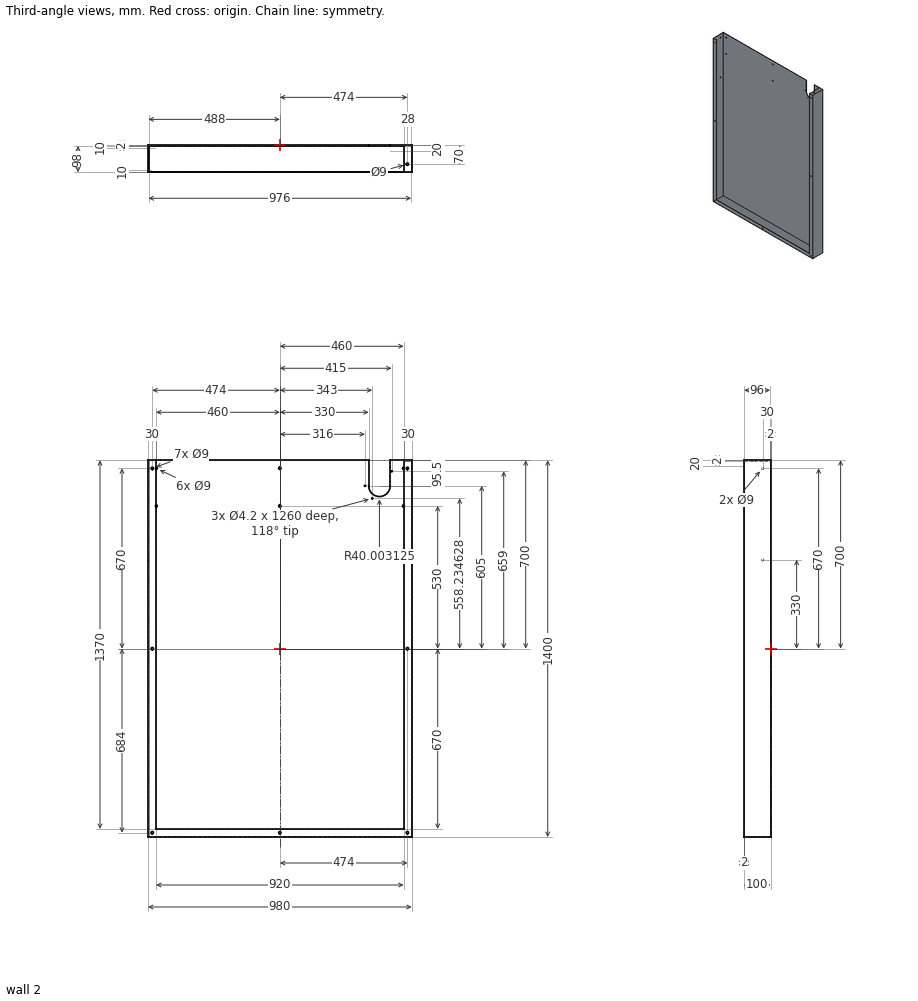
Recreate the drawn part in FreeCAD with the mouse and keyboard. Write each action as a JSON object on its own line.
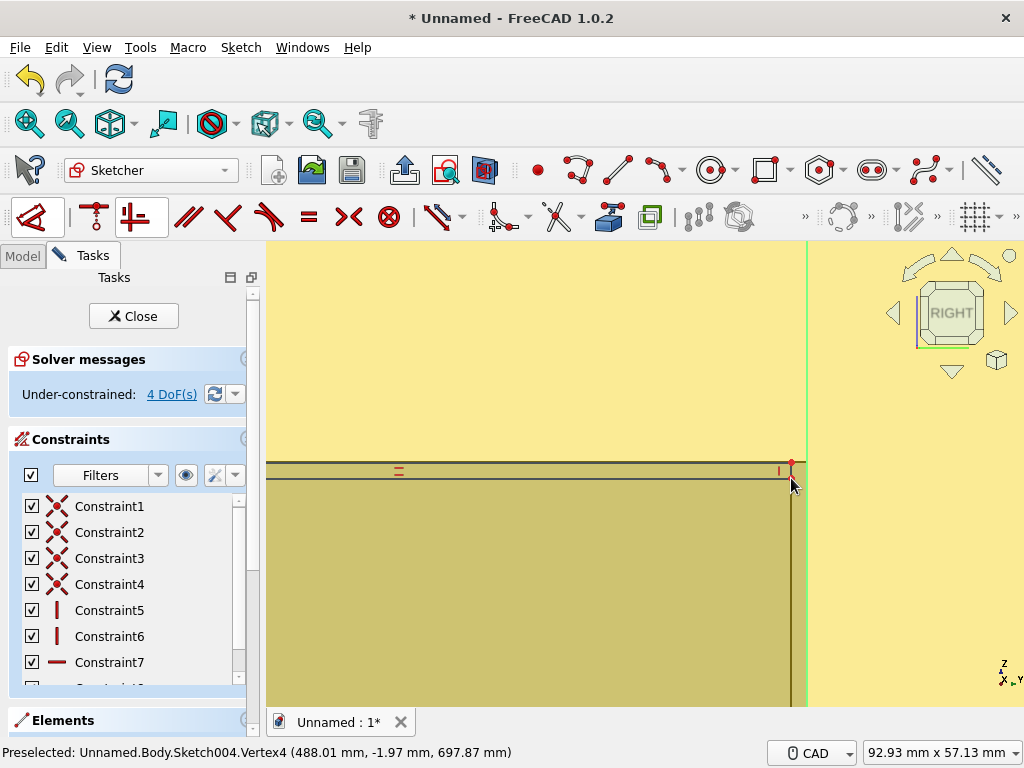
{"action": "scroll", "coordinate": [792, 479], "scroll_direction": "down", "scroll_amount": 3}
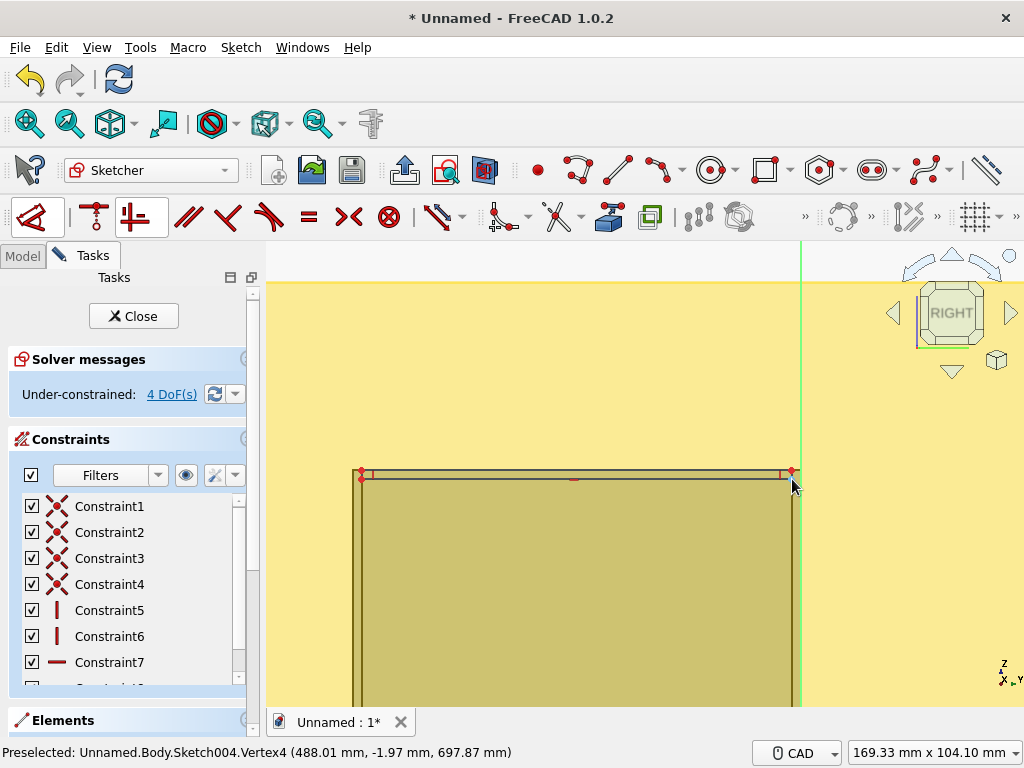
{"action": "scroll", "coordinate": [362, 475], "scroll_direction": "up", "scroll_amount": 8}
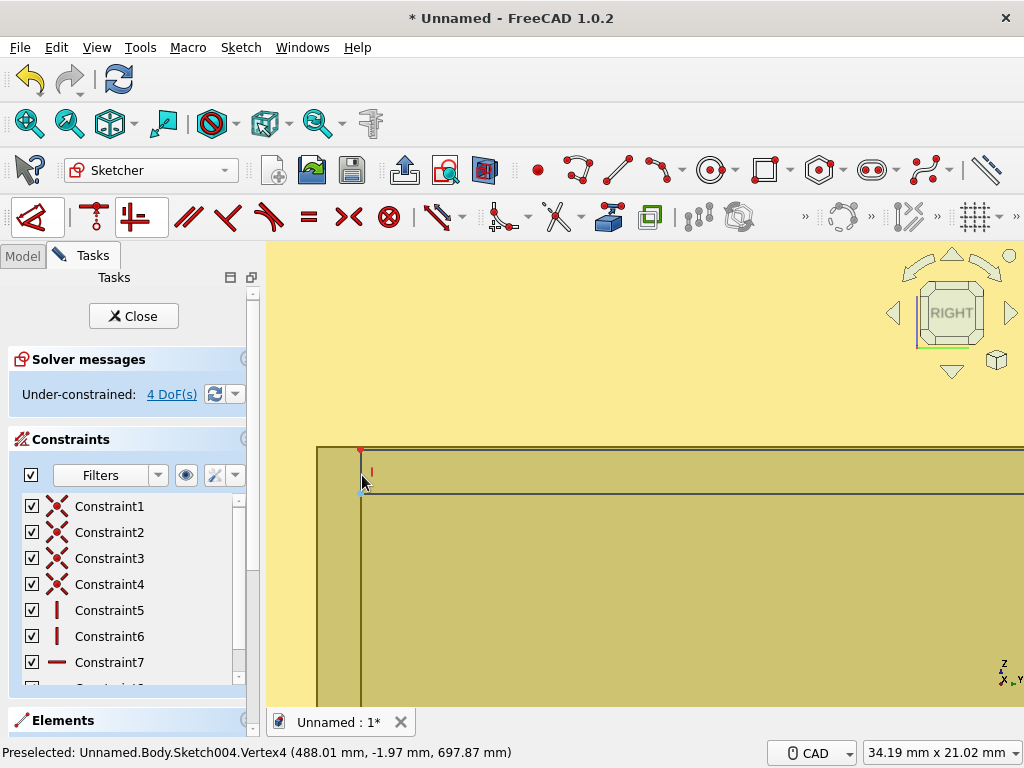
{"action": "left_click", "coordinate": [361, 472]}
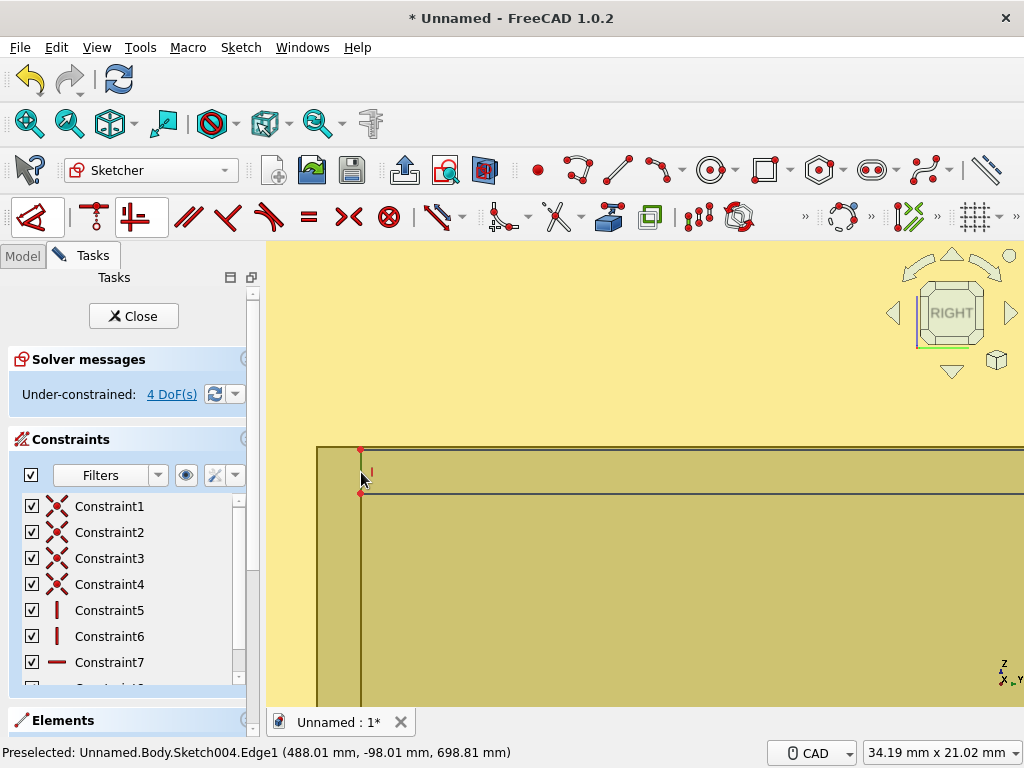
{"action": "left_click", "coordinate": [58, 218]}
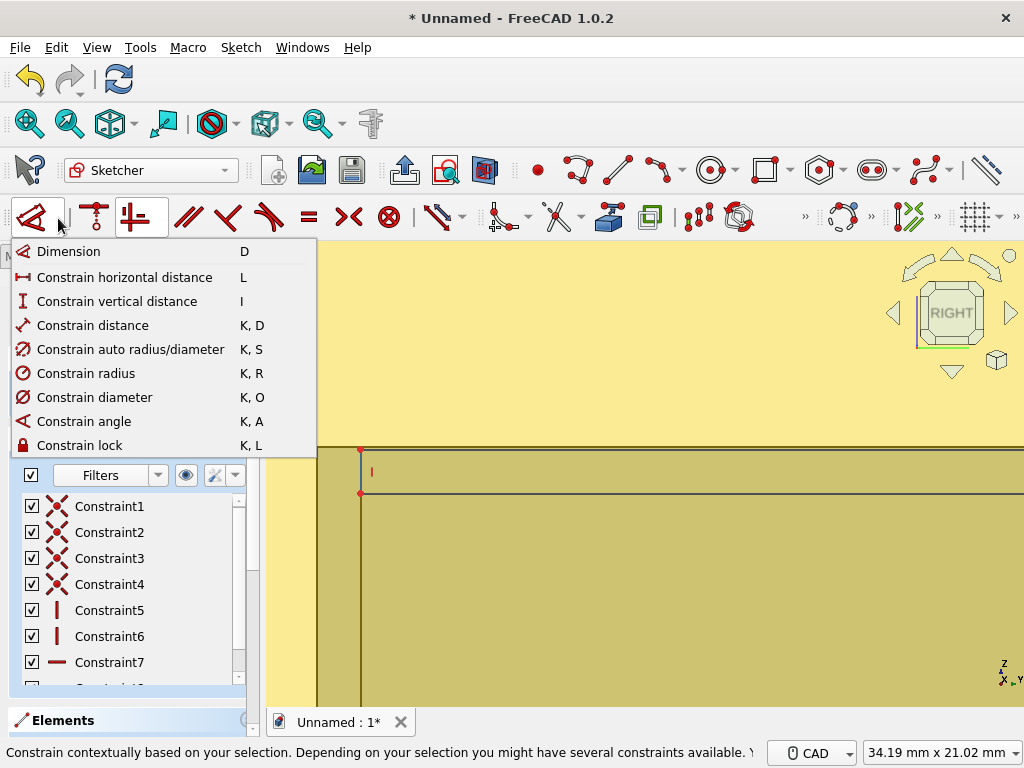
{"action": "left_click", "coordinate": [164, 301]}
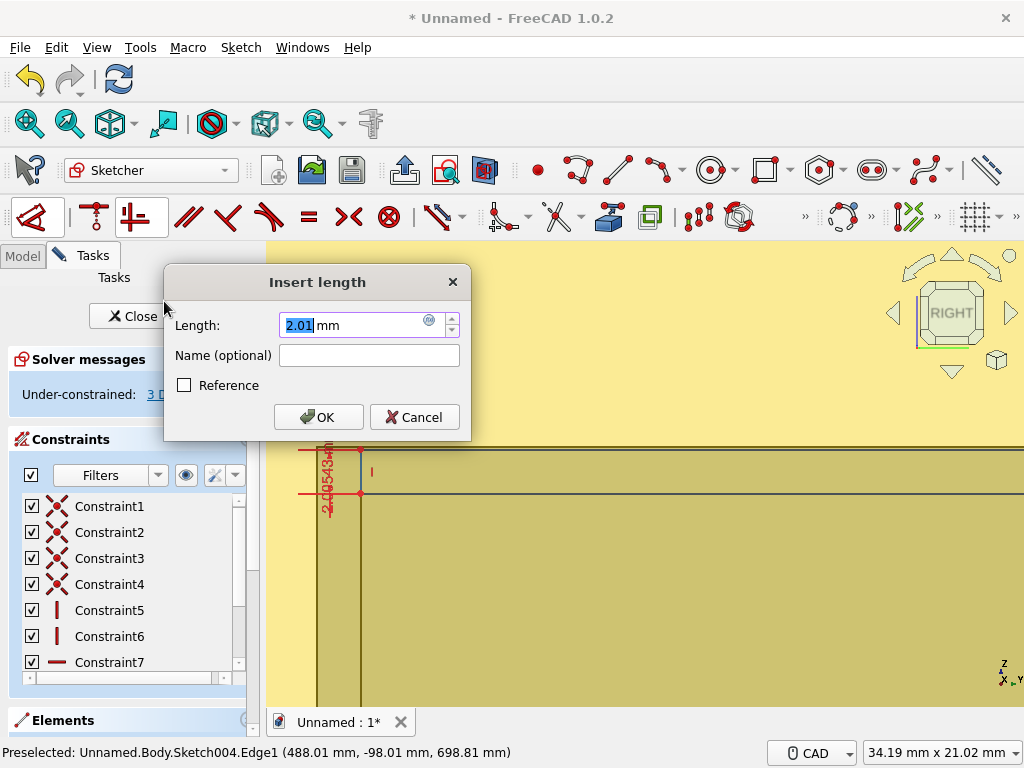
{"action": "type", "text": "2"}
{"action": "key", "text": "Return"}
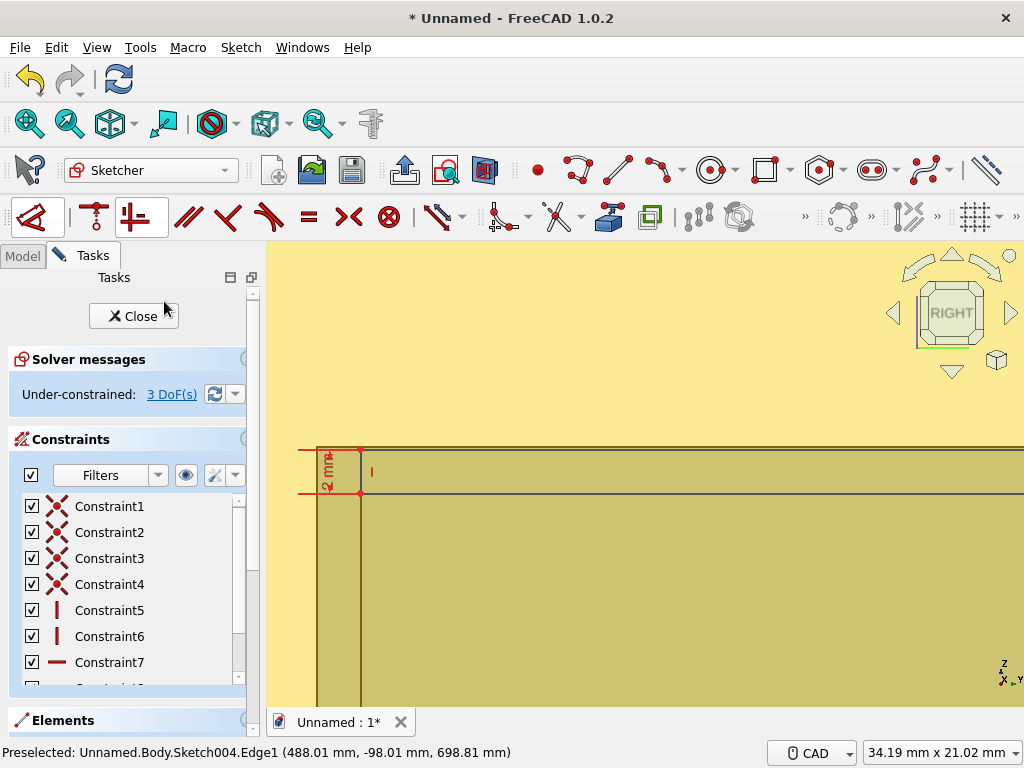
{"action": "scroll", "coordinate": [362, 475], "scroll_direction": "down", "scroll_amount": 8}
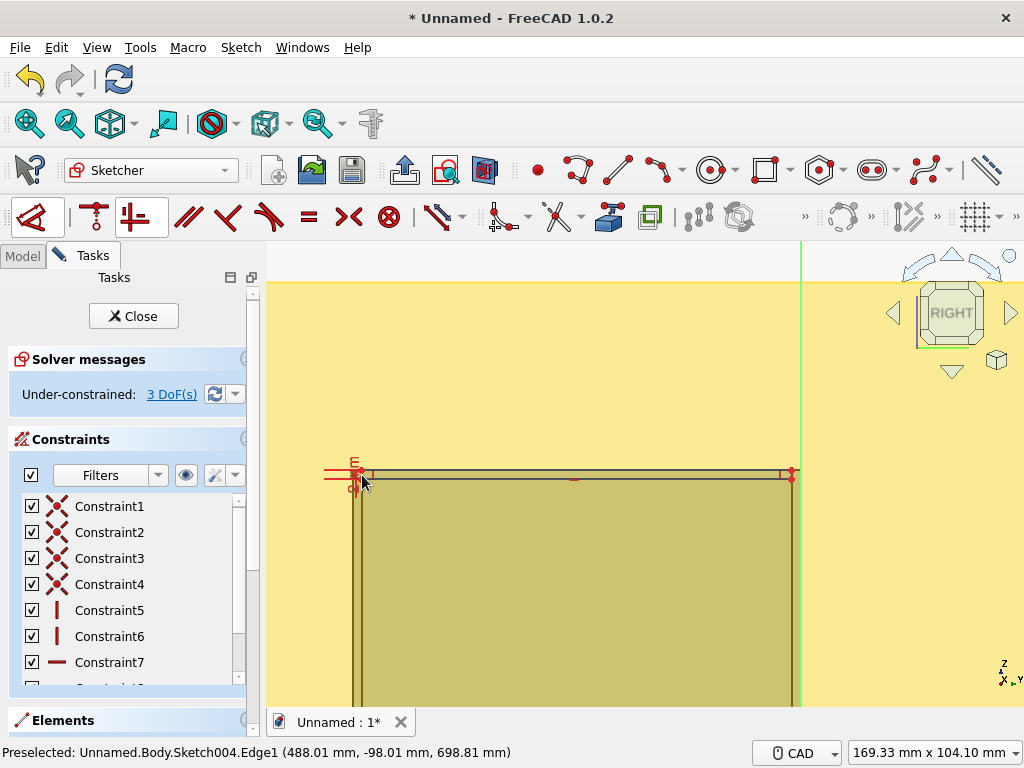
{"action": "scroll", "coordinate": [448, 479], "scroll_direction": "up", "scroll_amount": 3}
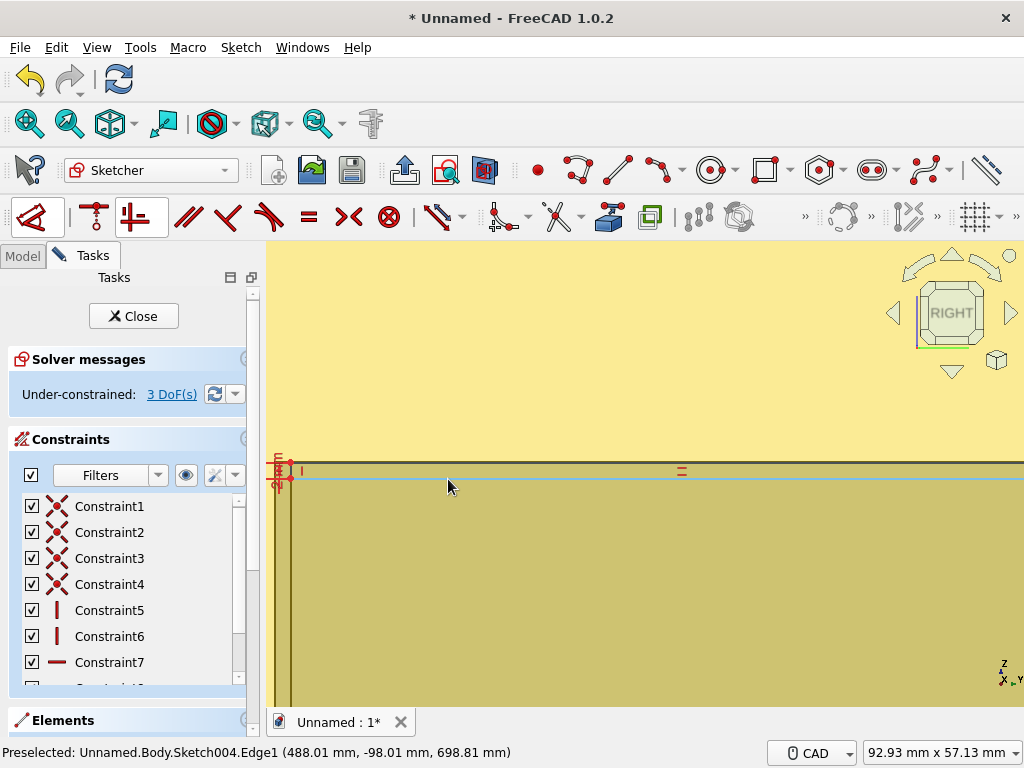
{"action": "left_click", "coordinate": [448, 479]}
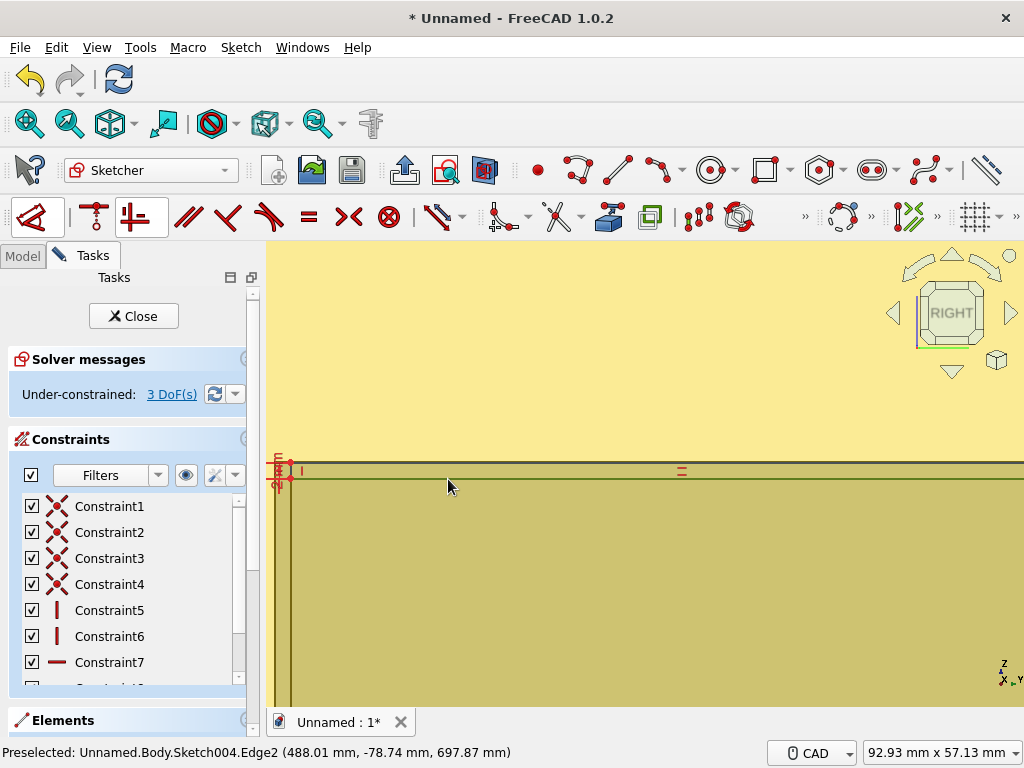
{"action": "left_click", "coordinate": [58, 218]}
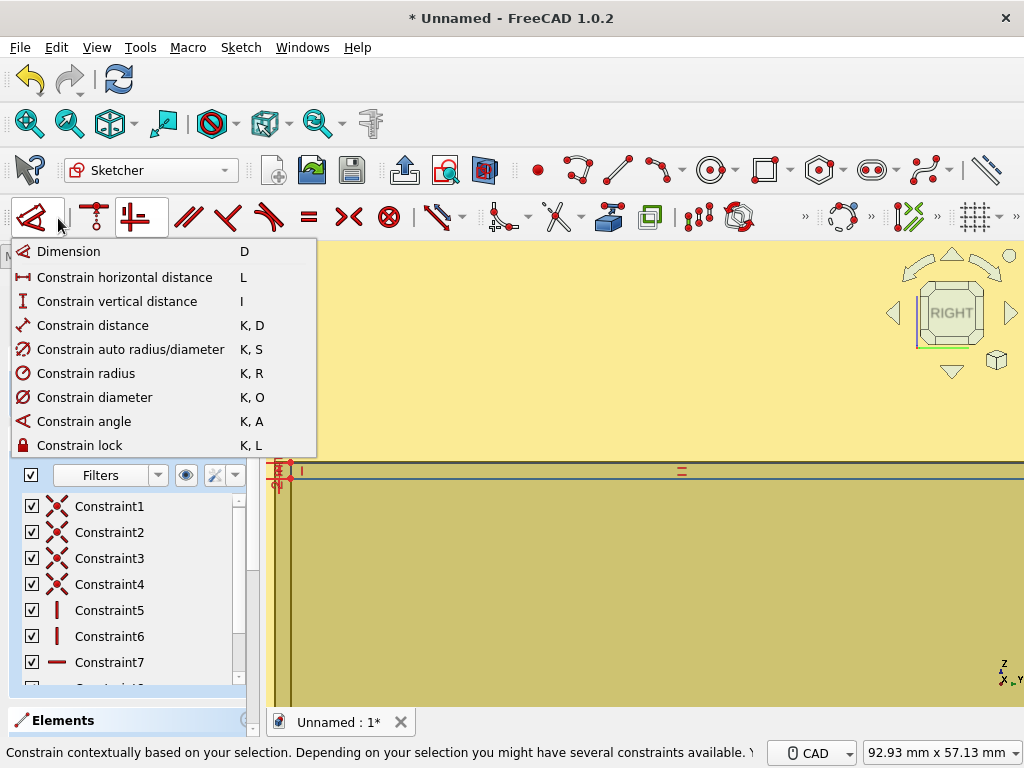
{"action": "left_click", "coordinate": [164, 277]}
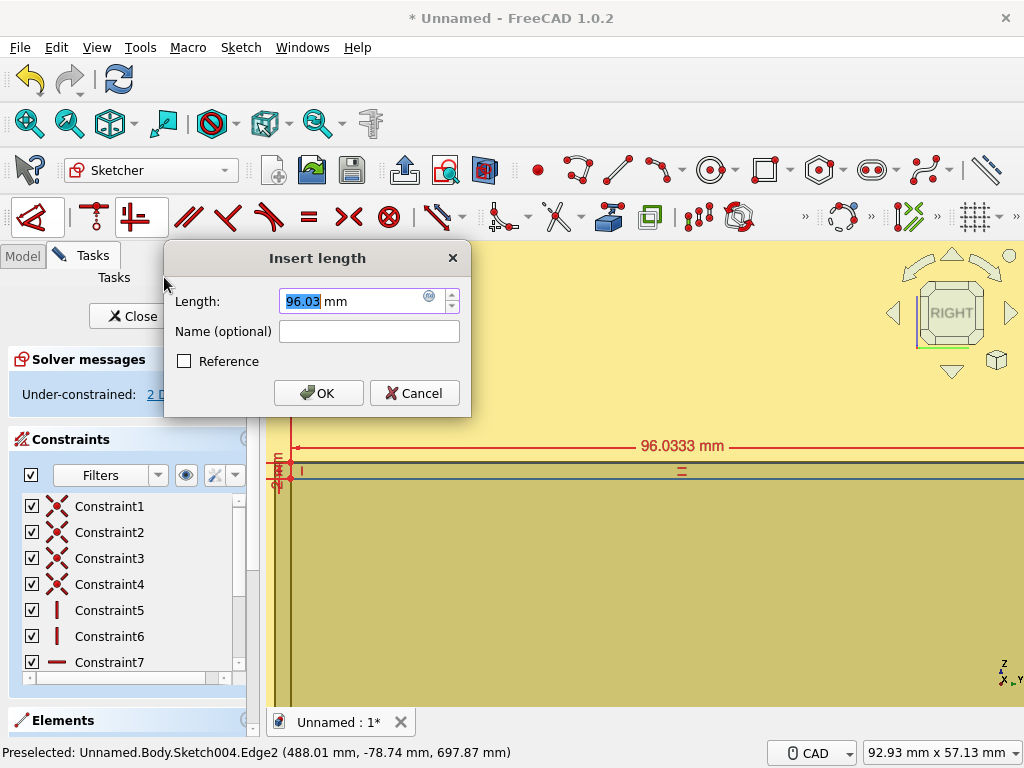
{"action": "type", "text": "96"}
{"action": "key", "text": "Return"}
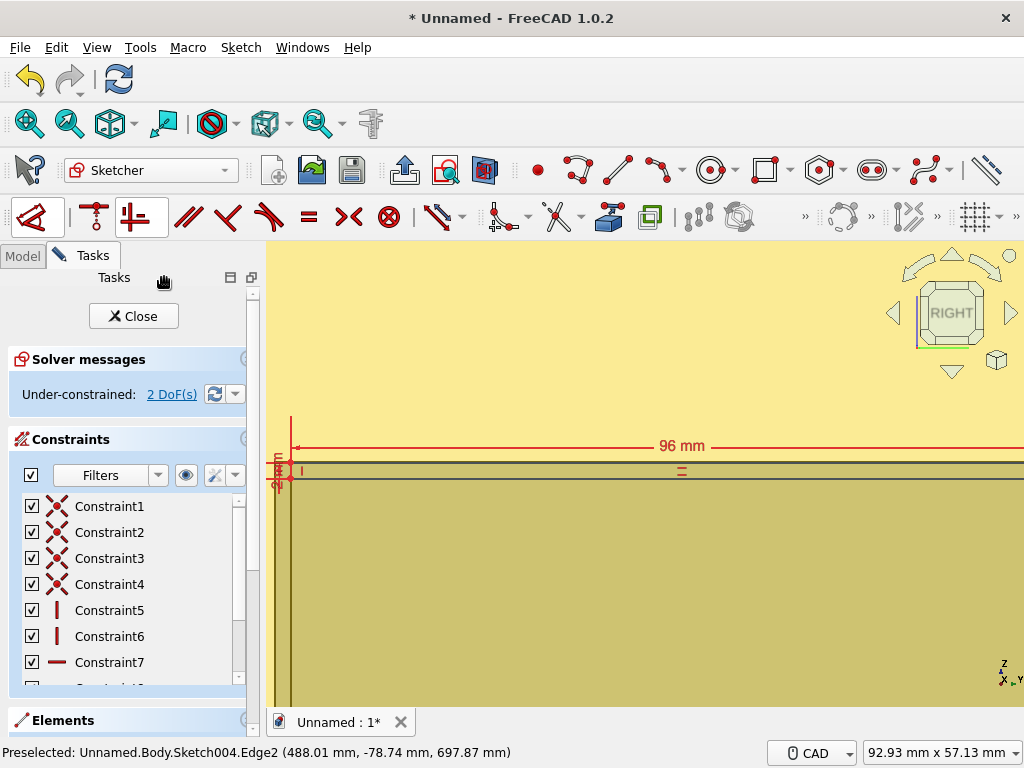
{"action": "scroll", "coordinate": [448, 479], "scroll_direction": "down", "scroll_amount": 3}